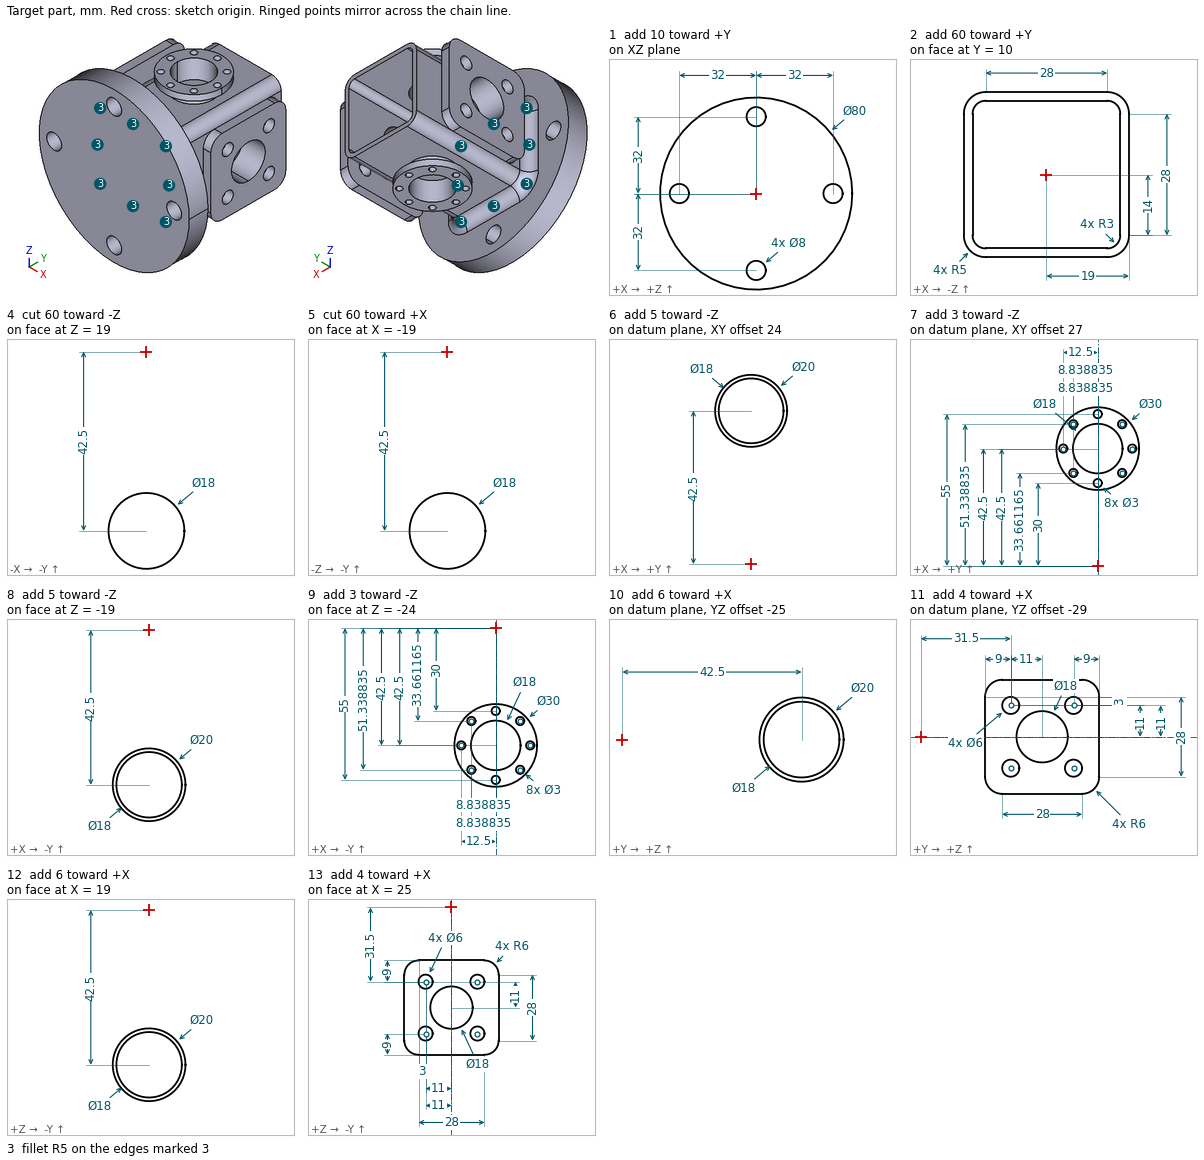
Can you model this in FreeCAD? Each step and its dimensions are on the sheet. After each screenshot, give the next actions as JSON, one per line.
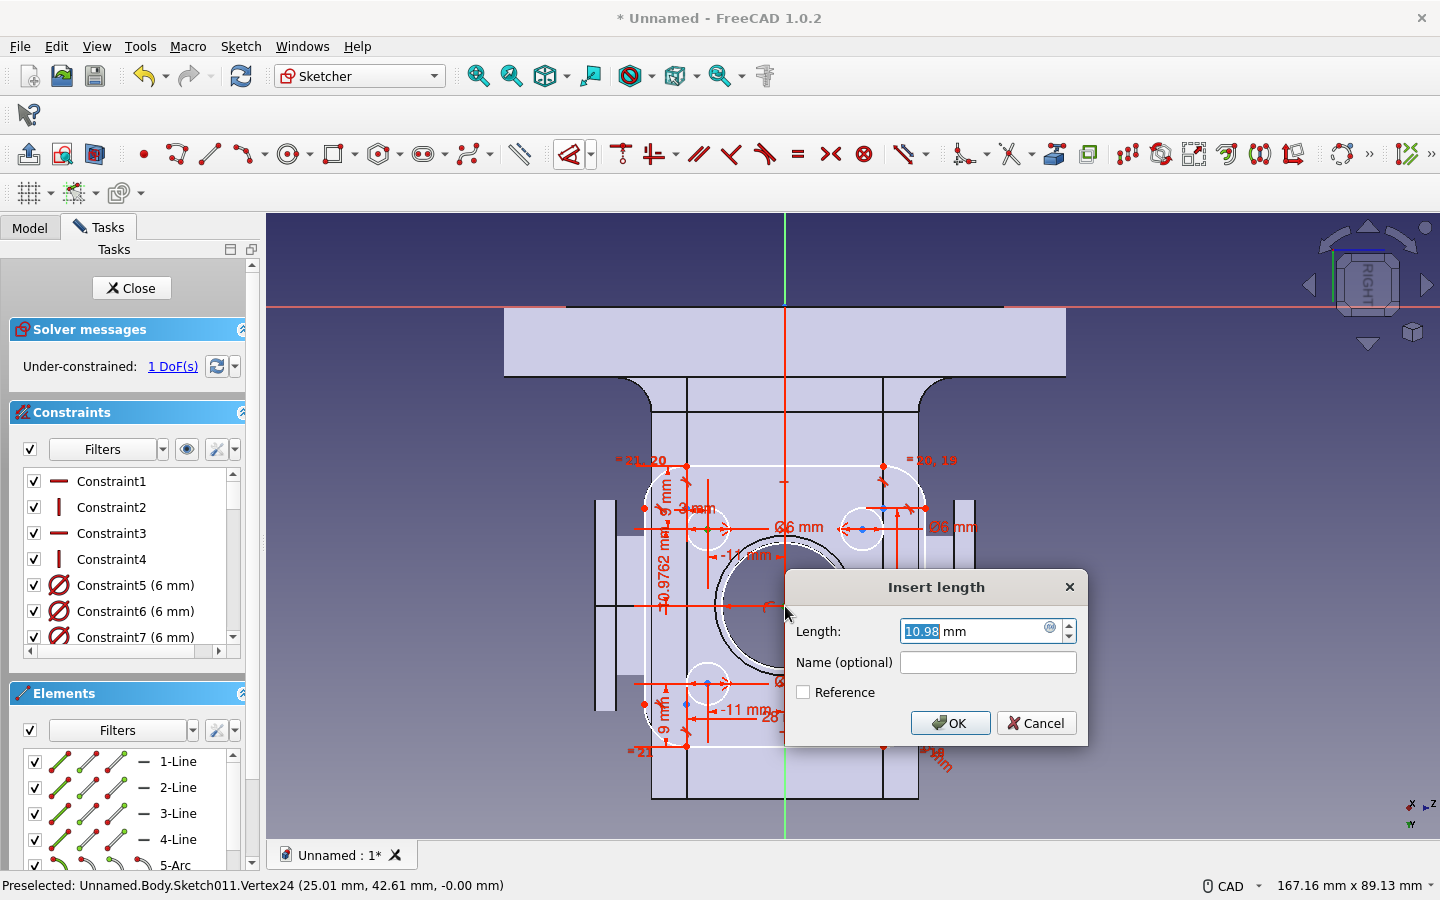
{"action": "type", "text": "11"}
{"action": "key", "text": "Return"}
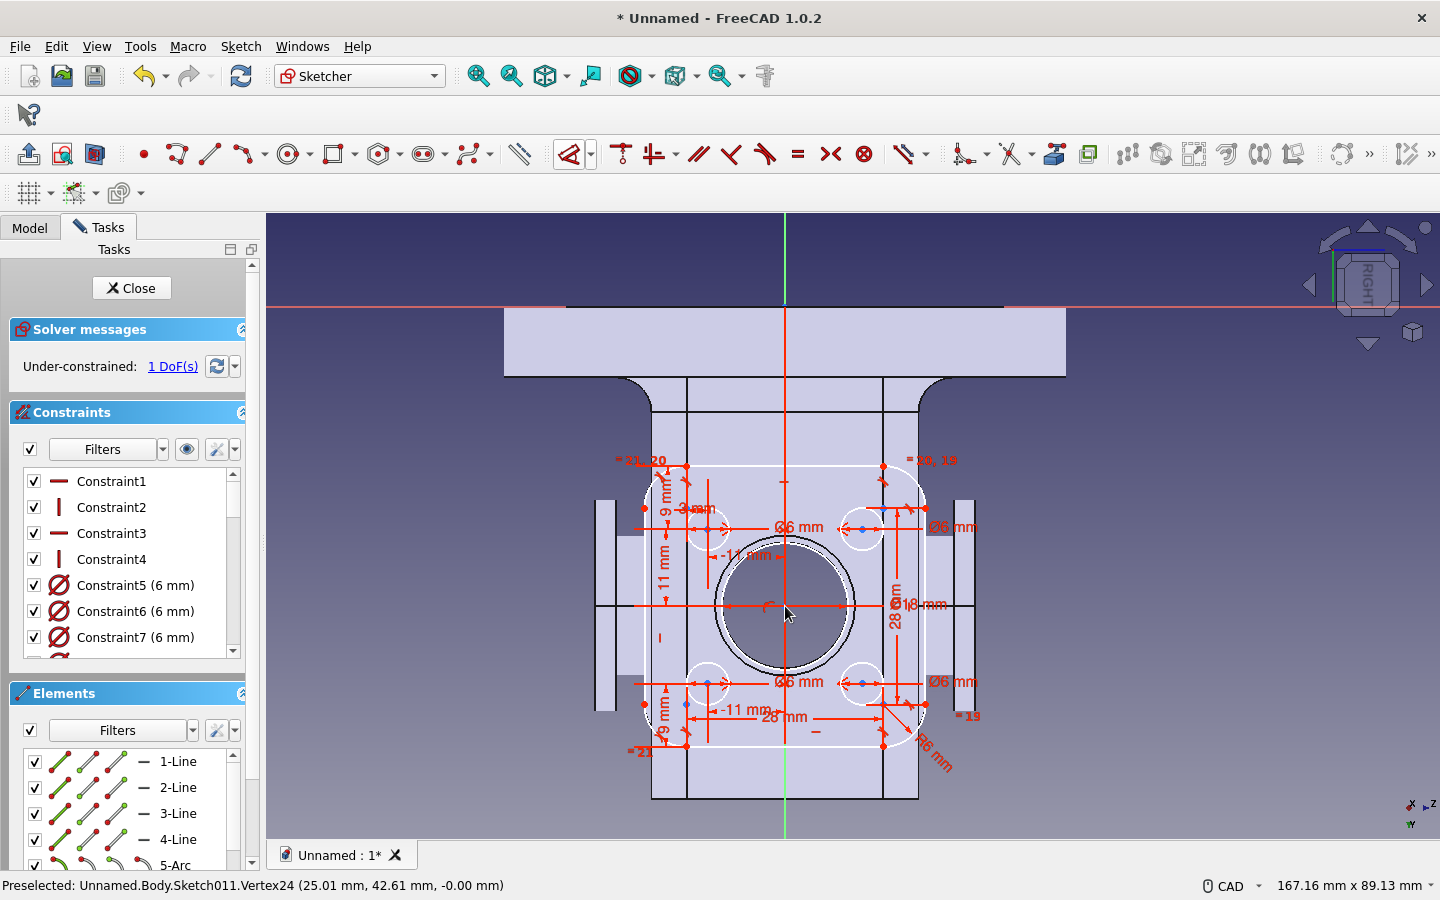
{"action": "left_click", "coordinate": [708, 529]}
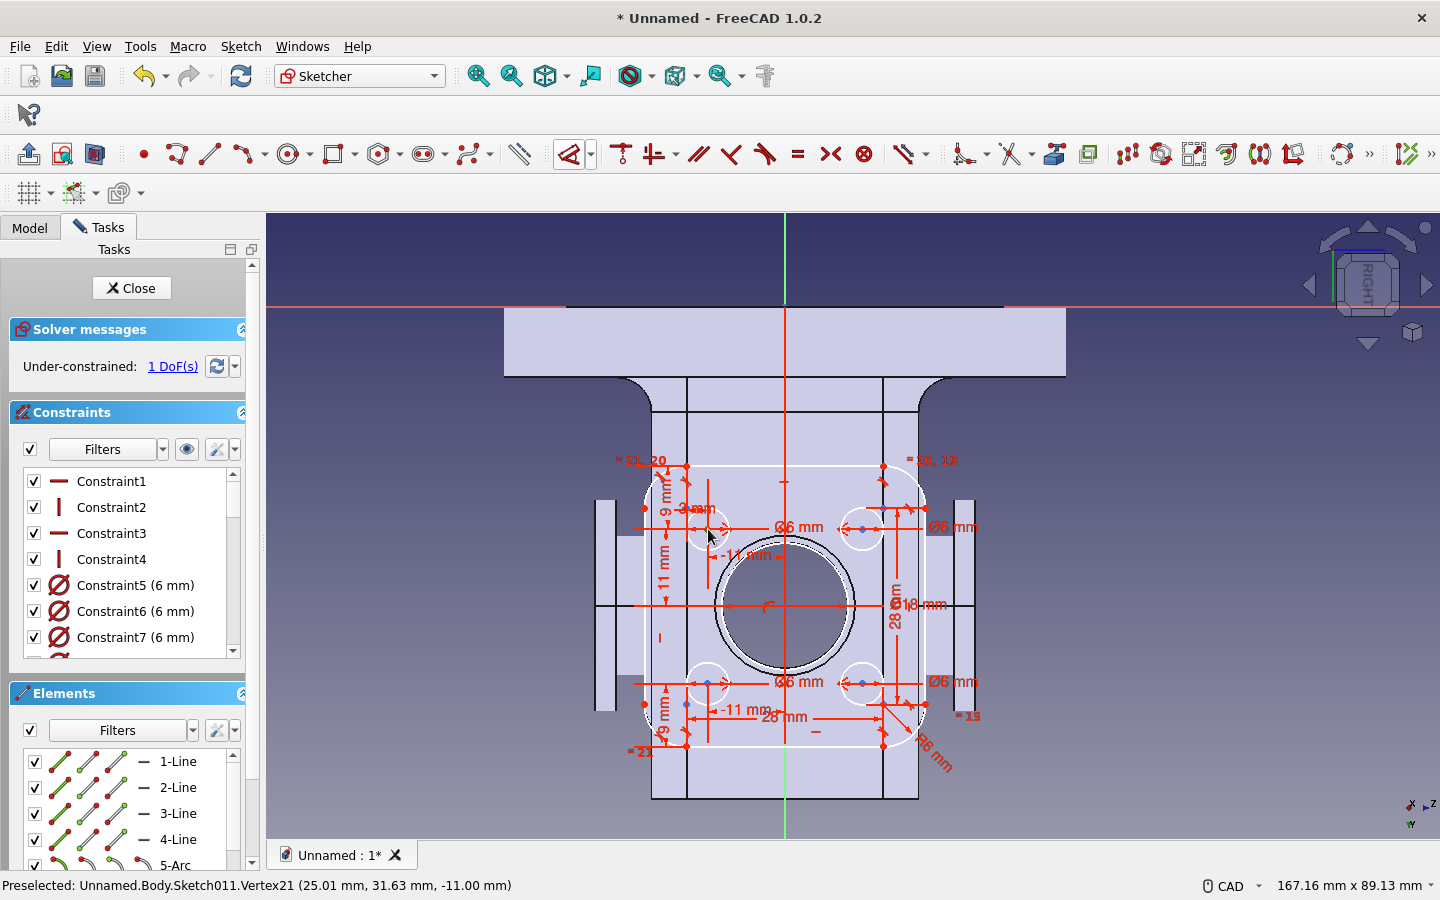
{"action": "left_click", "coordinate": [590, 154]}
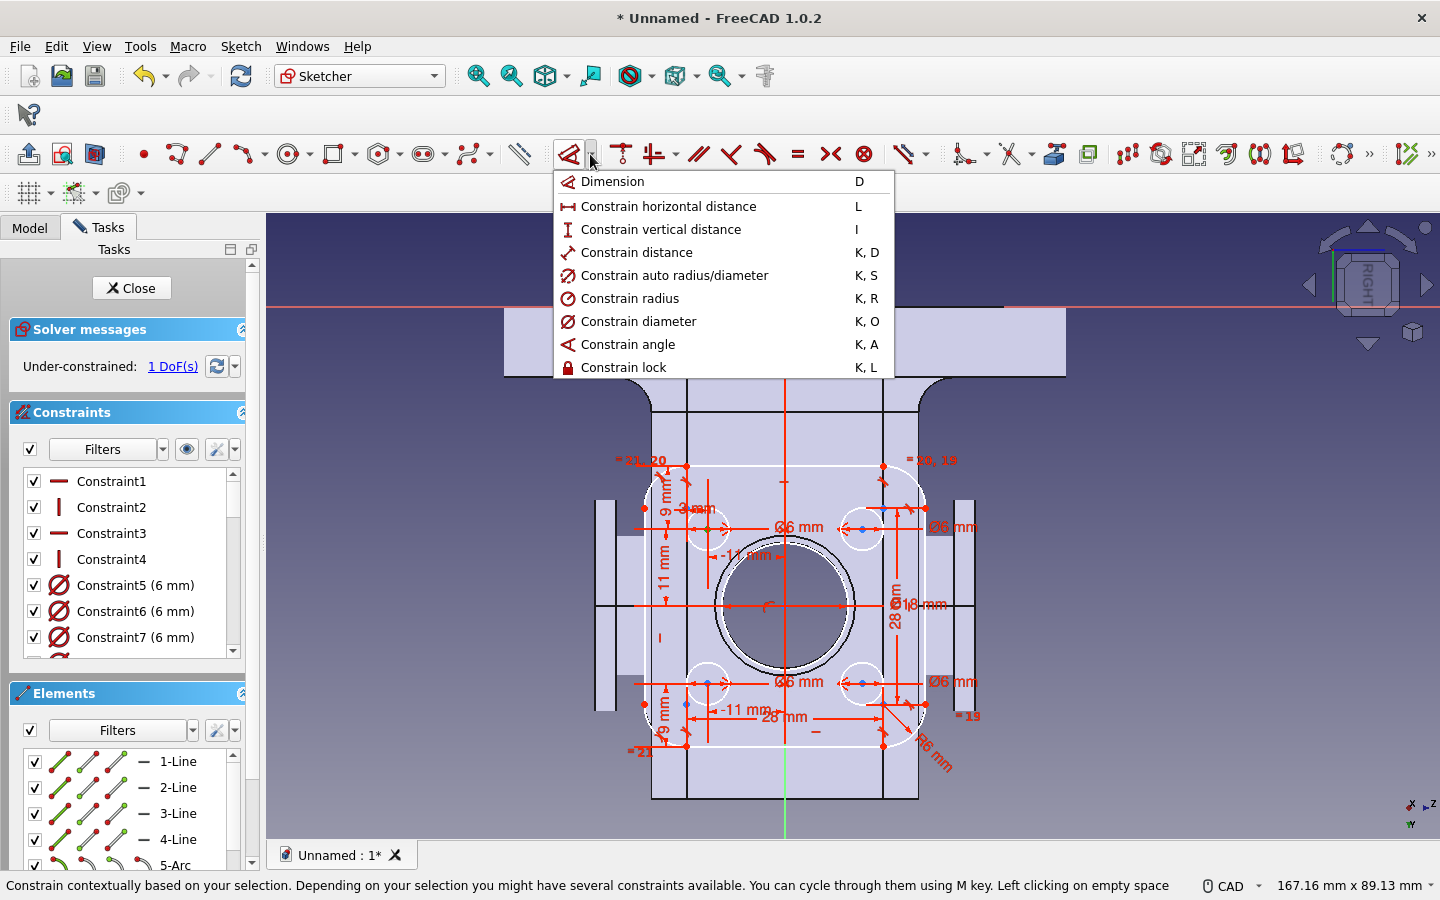
{"action": "left_click", "coordinate": [724, 230]}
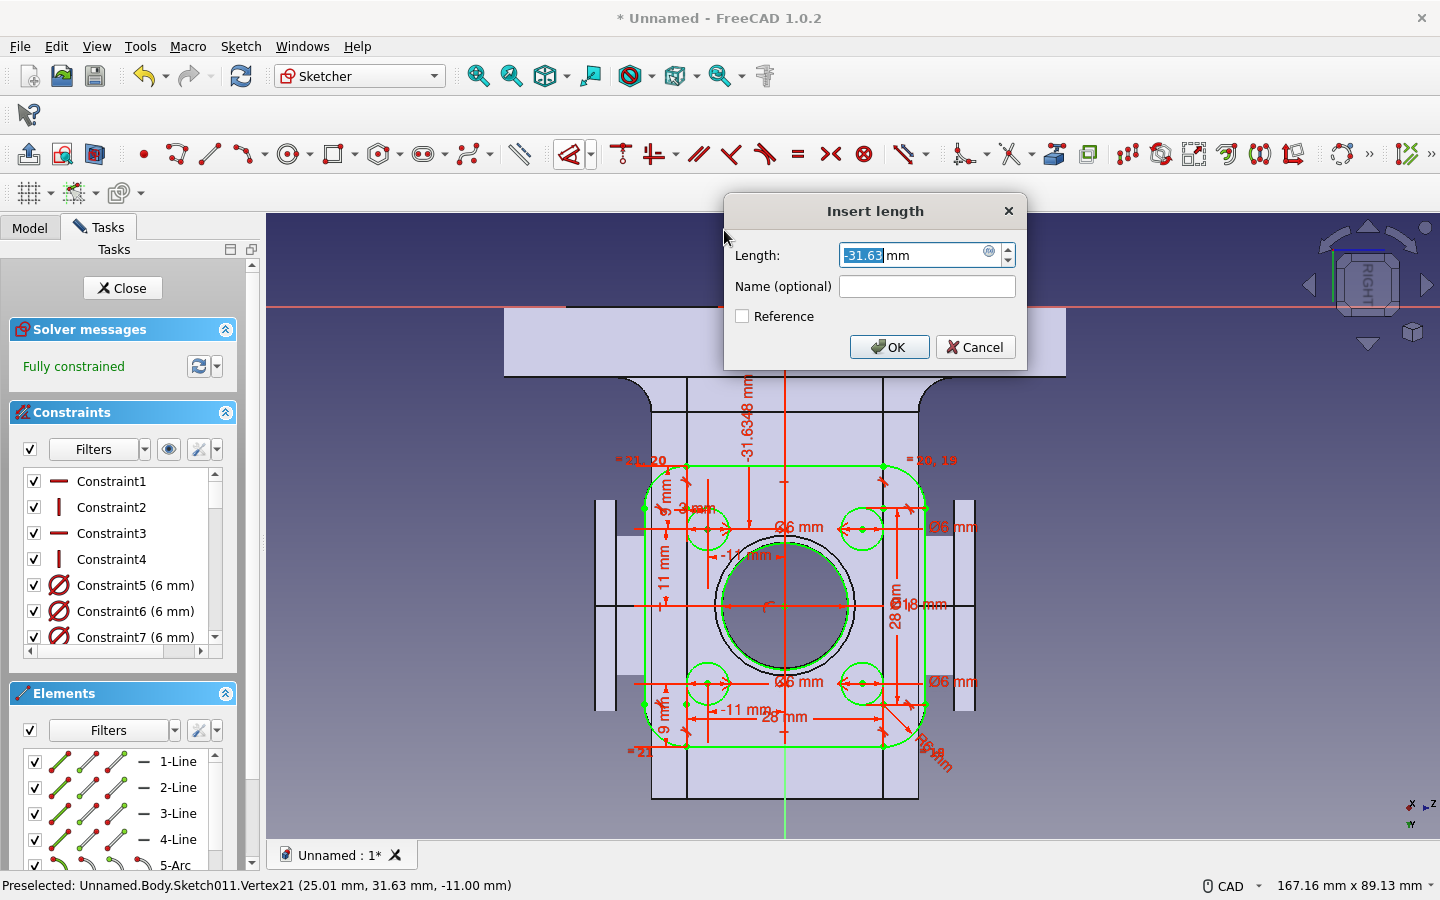
{"action": "type", "text": "-31.5"}
{"action": "key", "text": "Return"}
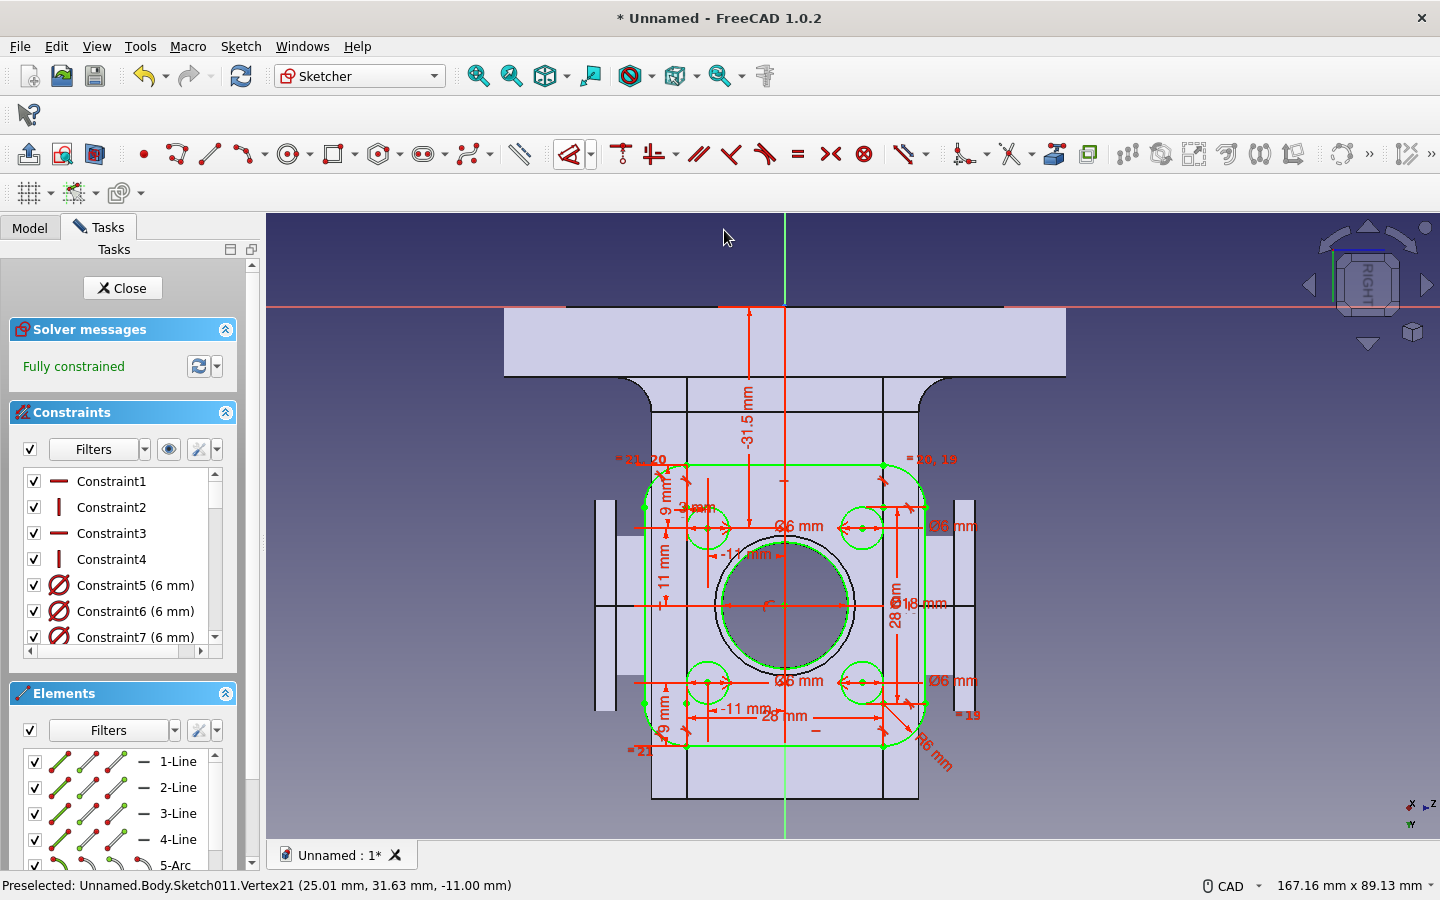
{"action": "left_click", "coordinate": [123, 288]}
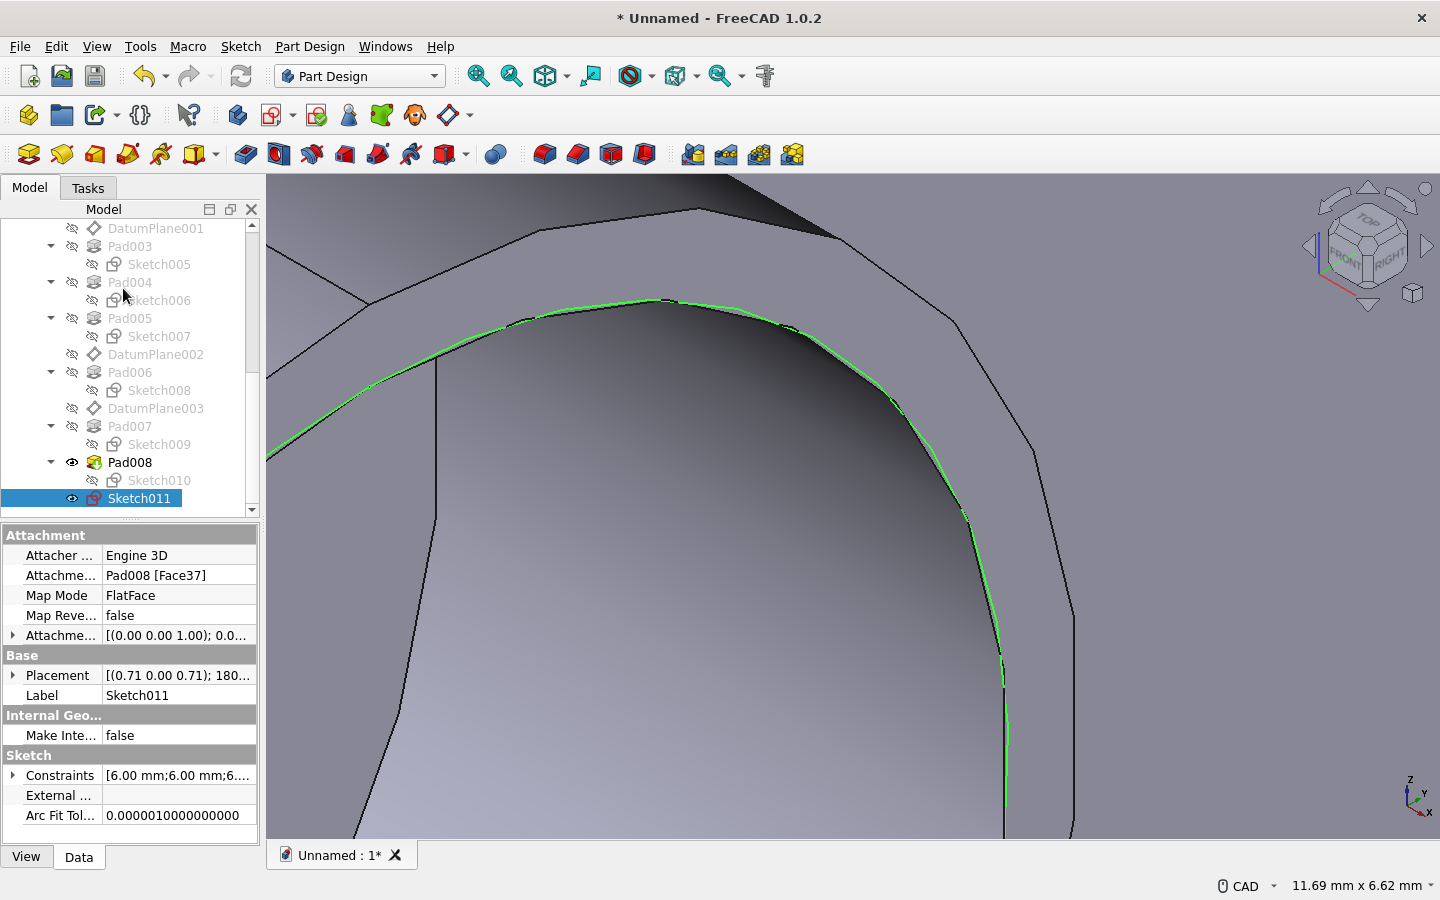
{"action": "left_click", "coordinate": [29, 154]}